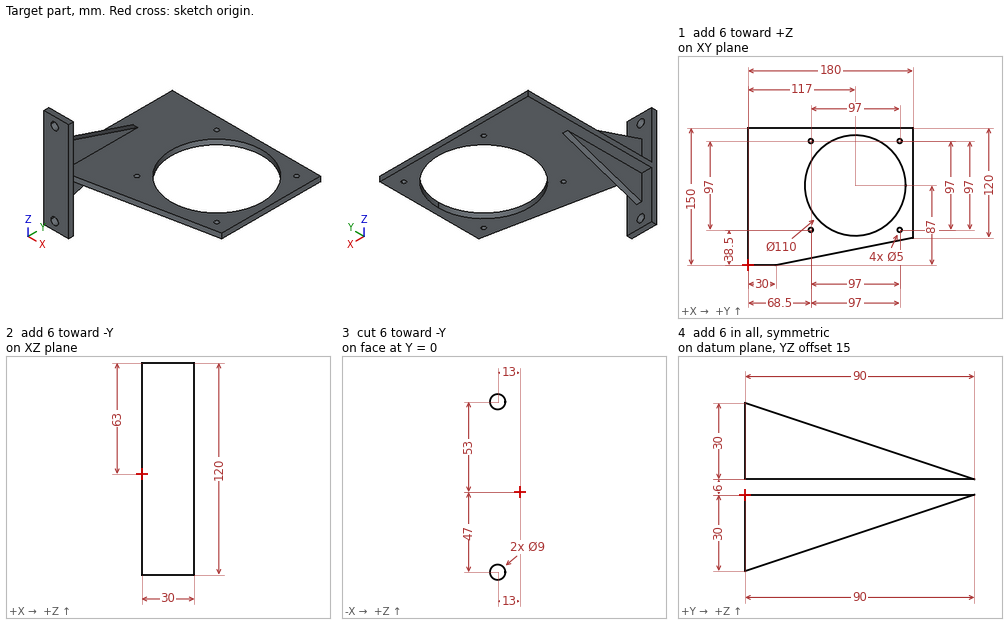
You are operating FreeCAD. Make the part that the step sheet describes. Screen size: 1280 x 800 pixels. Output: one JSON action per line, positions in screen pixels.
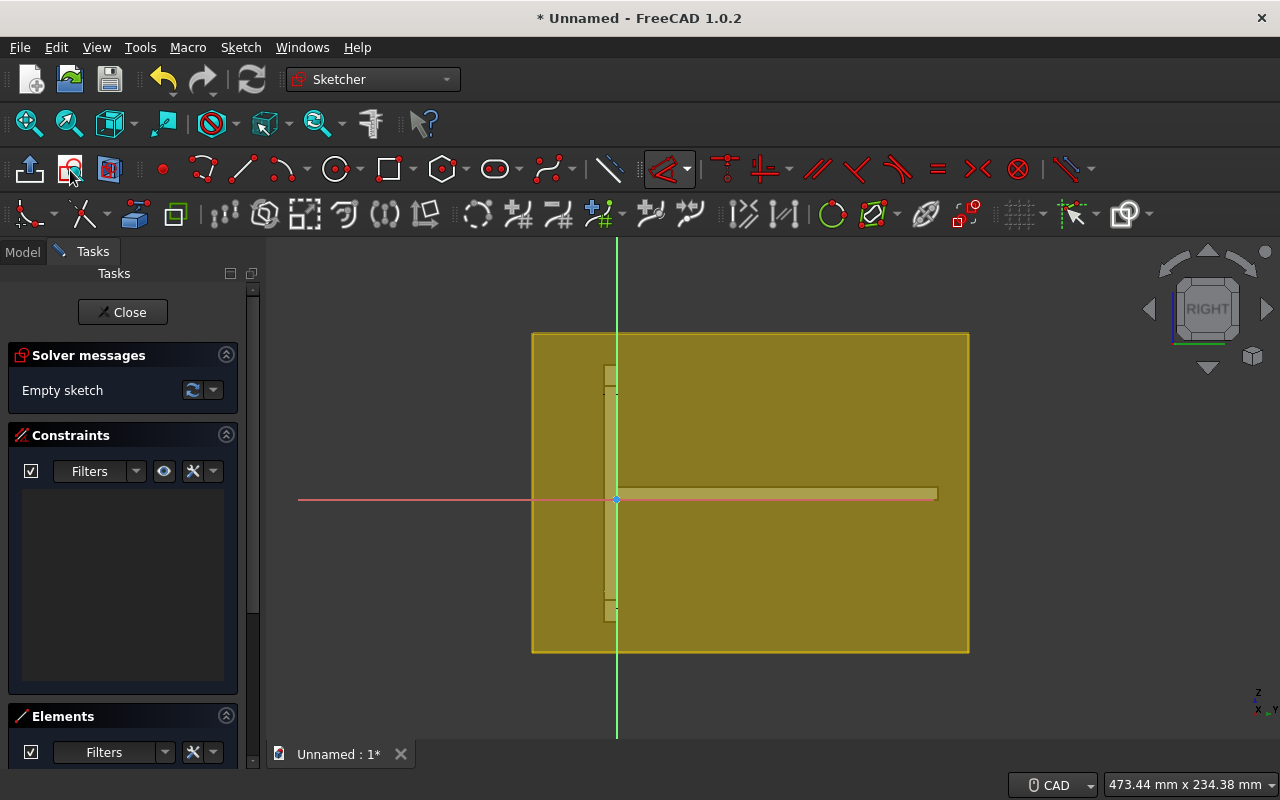
{"action": "scroll", "coordinate": [720, 497], "scroll_direction": "up", "scroll_amount": 4}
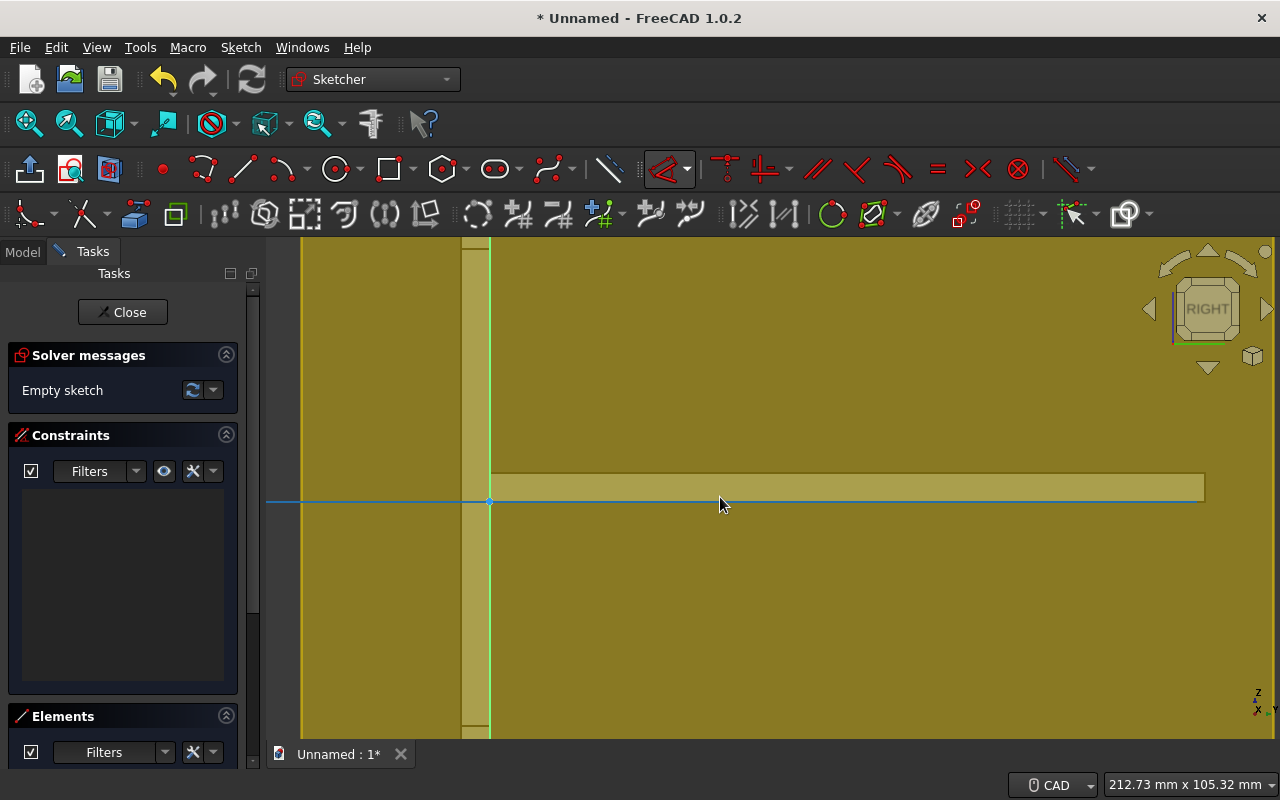
{"action": "key", "text": "g m"}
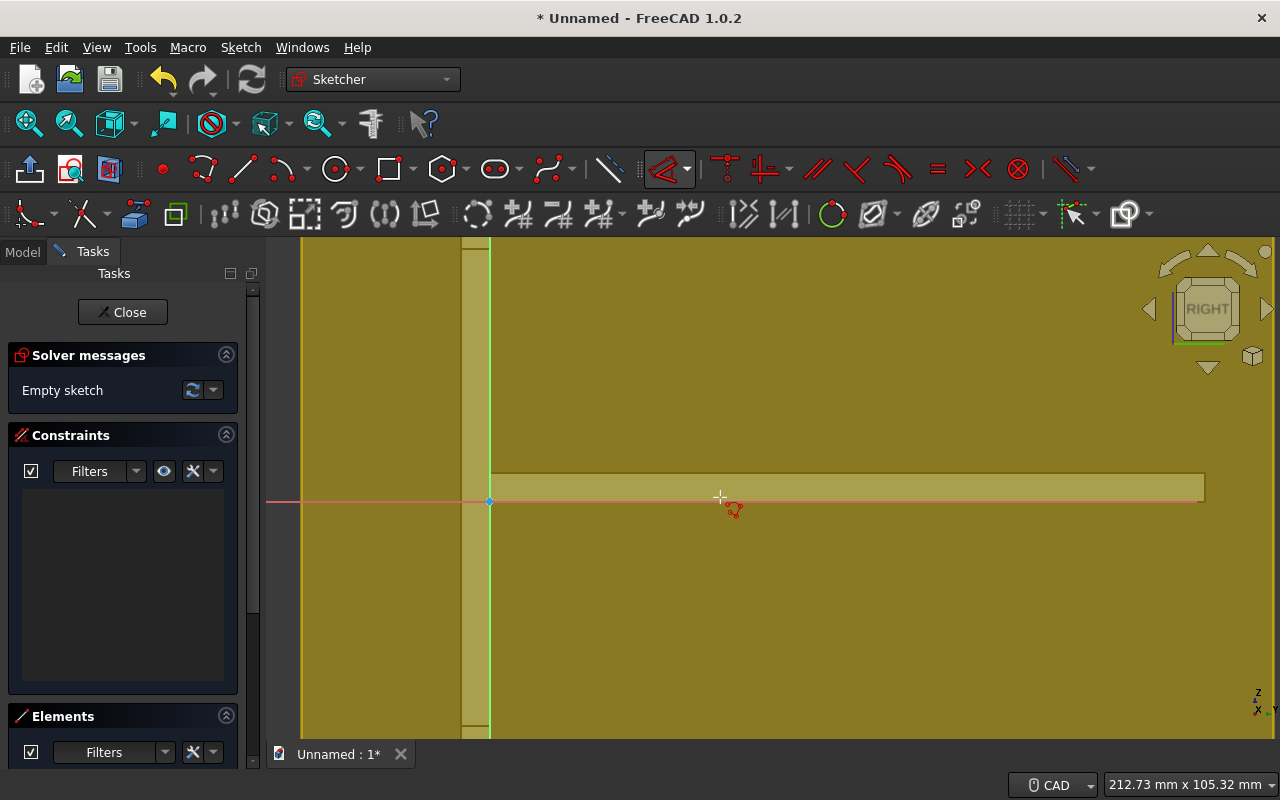
{"action": "left_click", "coordinate": [490, 502]}
{"action": "left_click", "coordinate": [919, 493]}
{"action": "left_click", "coordinate": [499, 645]}
{"action": "left_click", "coordinate": [490, 502]}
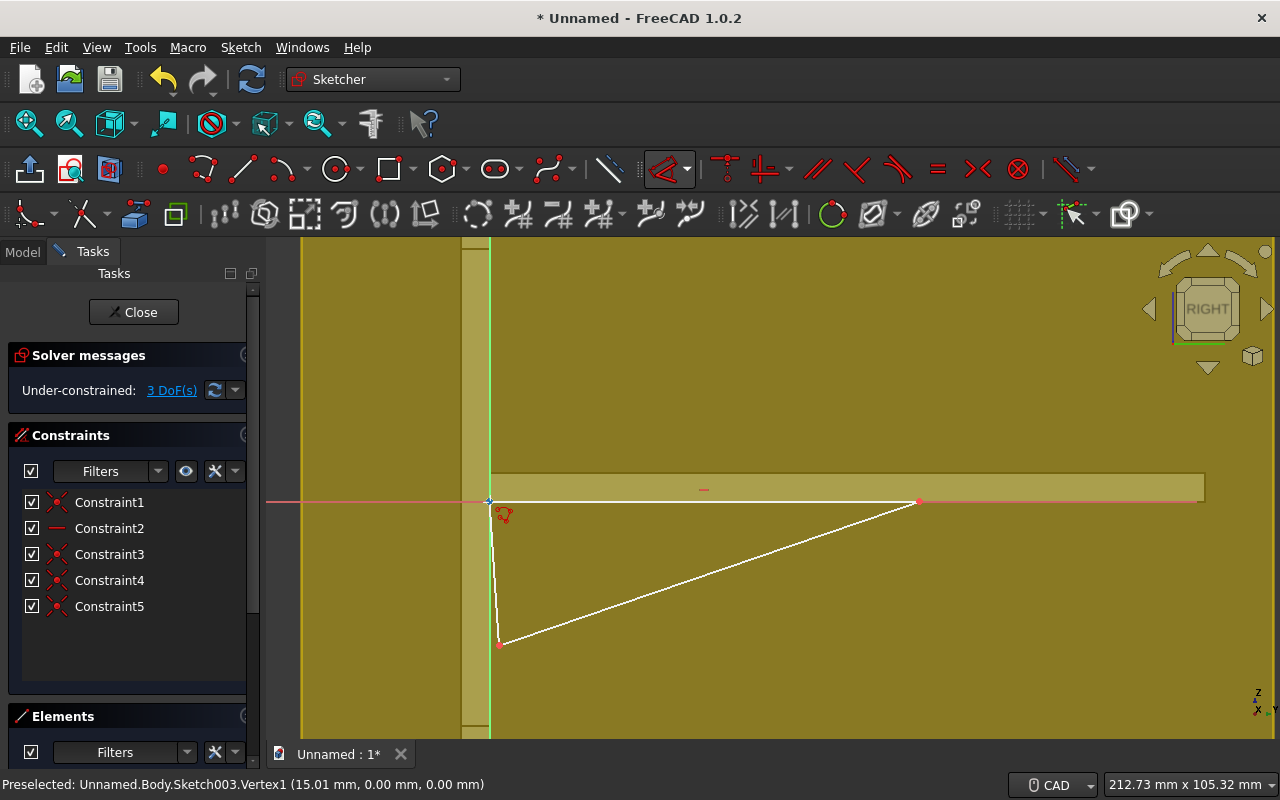
{"action": "left_click", "coordinate": [490, 473]}
{"action": "left_click", "coordinate": [499, 330]}
{"action": "left_click", "coordinate": [919, 473]}
{"action": "left_click", "coordinate": [490, 474]}
{"action": "key", "text": "Escape"}
{"action": "key", "text": "Escape"}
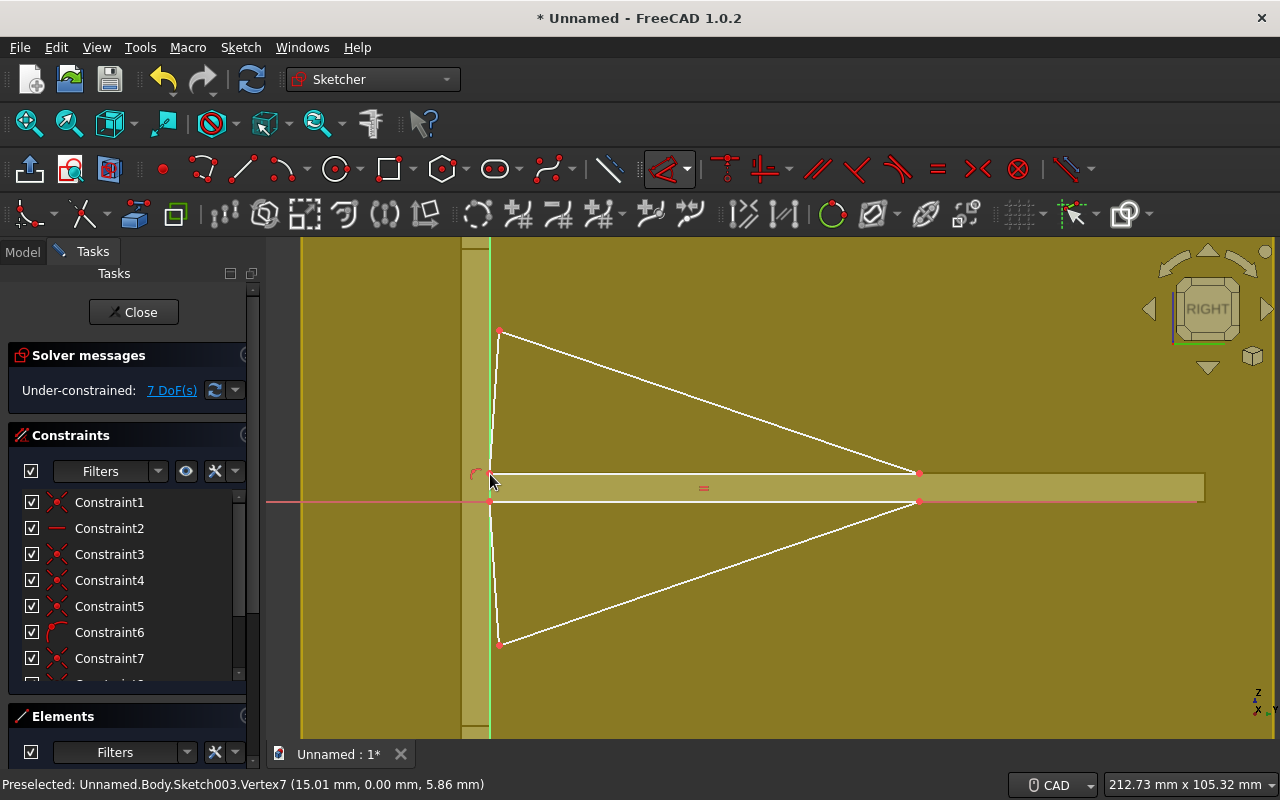
{"action": "left_click", "coordinate": [492, 545]}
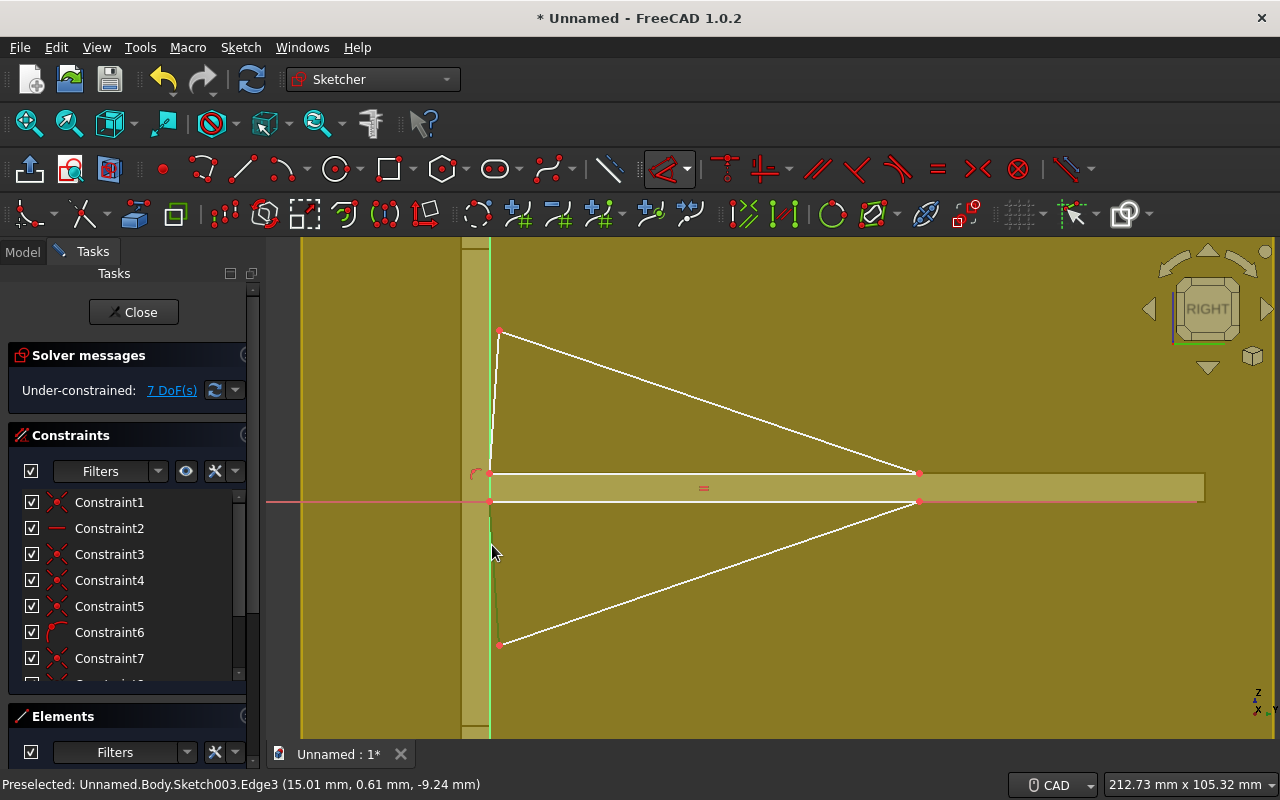
{"action": "key", "text": "v"}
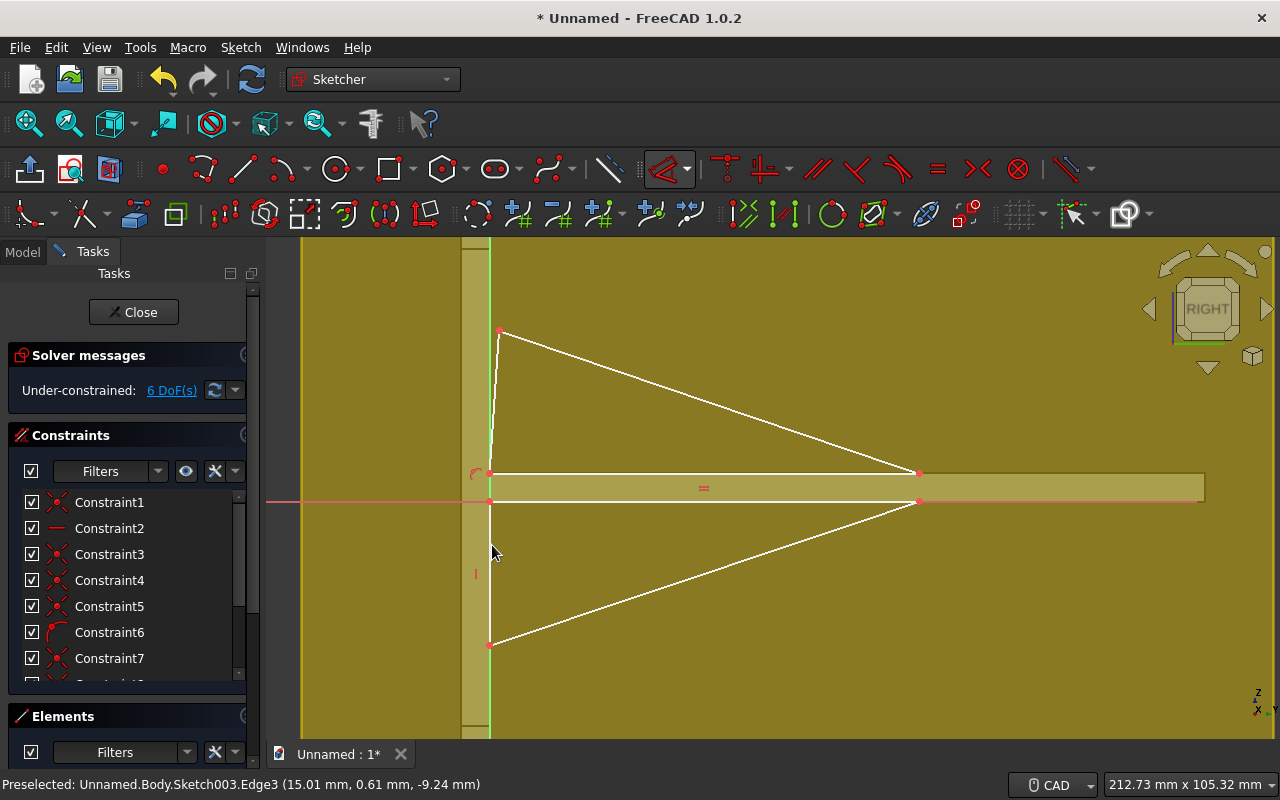
{"action": "left_click", "coordinate": [492, 431]}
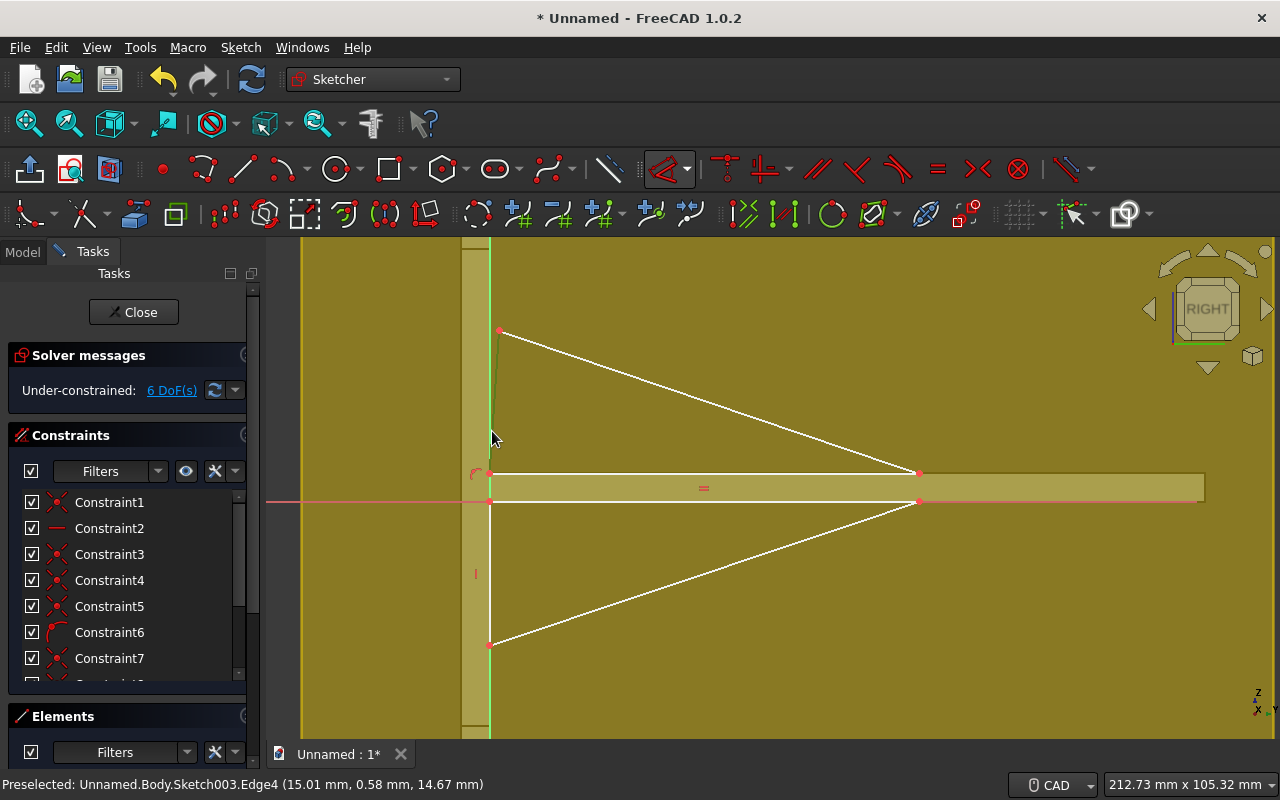
{"action": "key", "text": "v"}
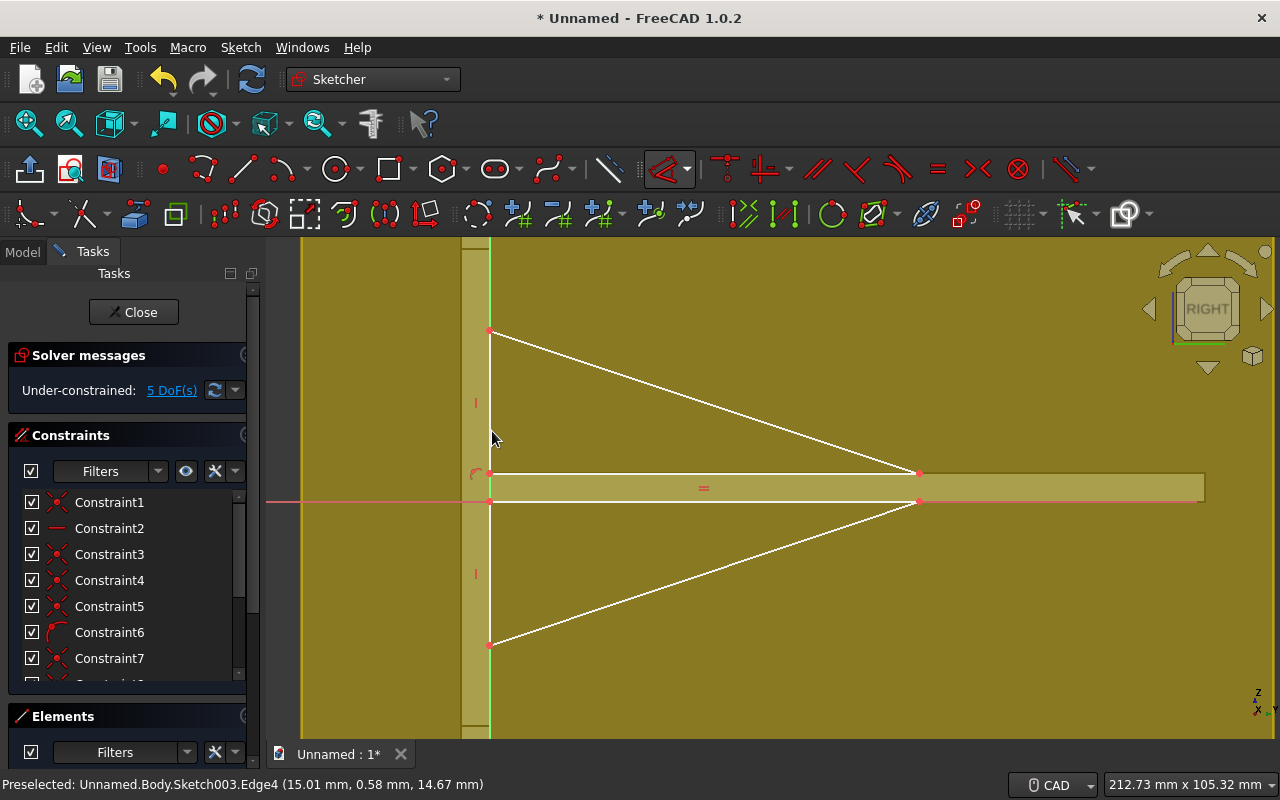
{"action": "left_click", "coordinate": [618, 502]}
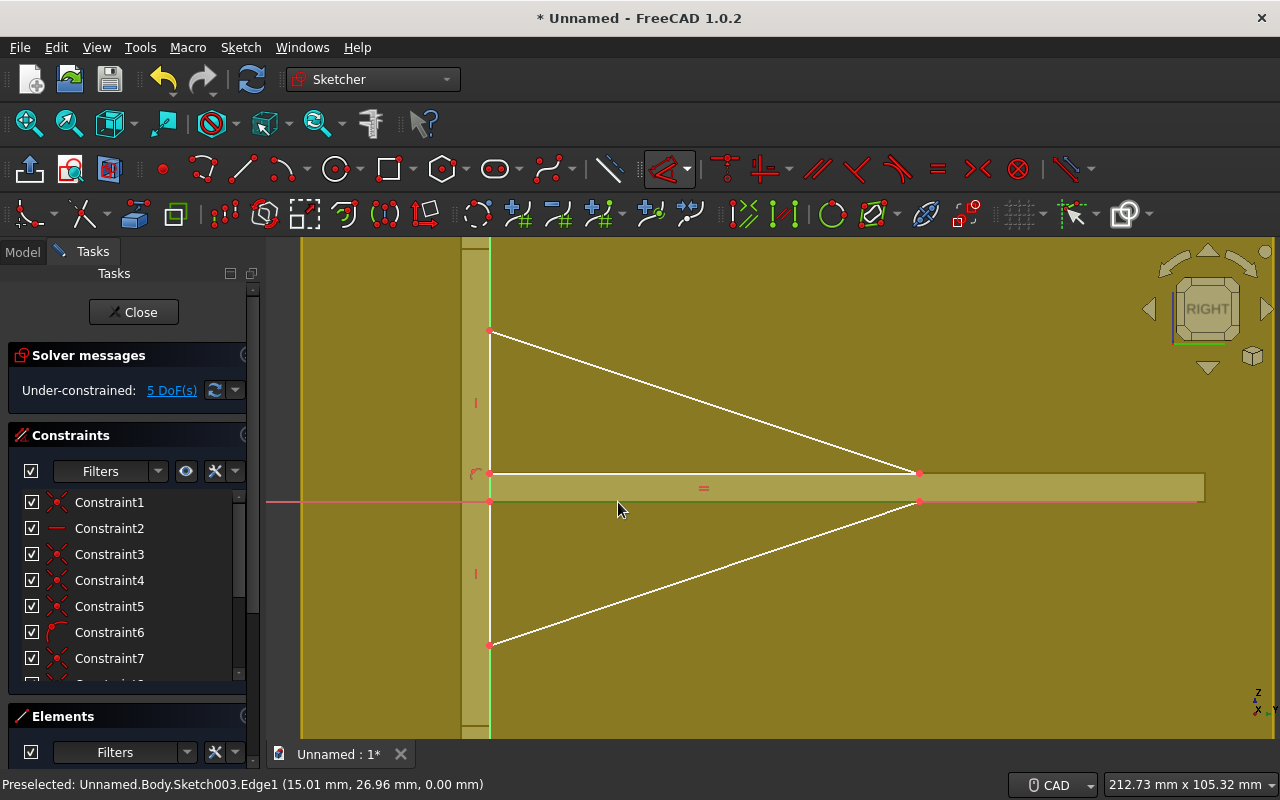
{"action": "key", "text": "l"}